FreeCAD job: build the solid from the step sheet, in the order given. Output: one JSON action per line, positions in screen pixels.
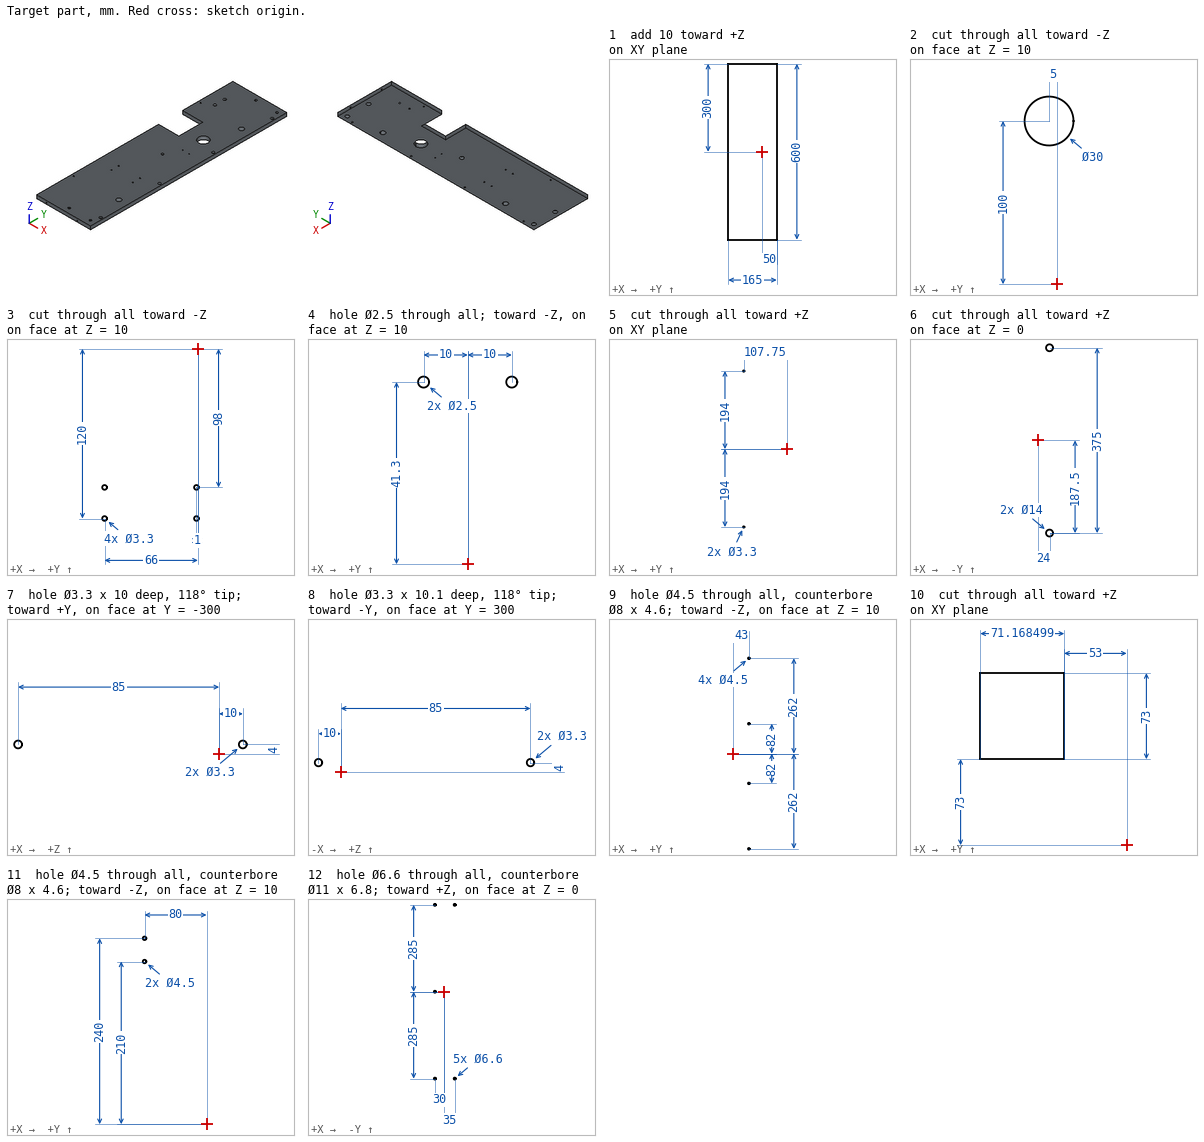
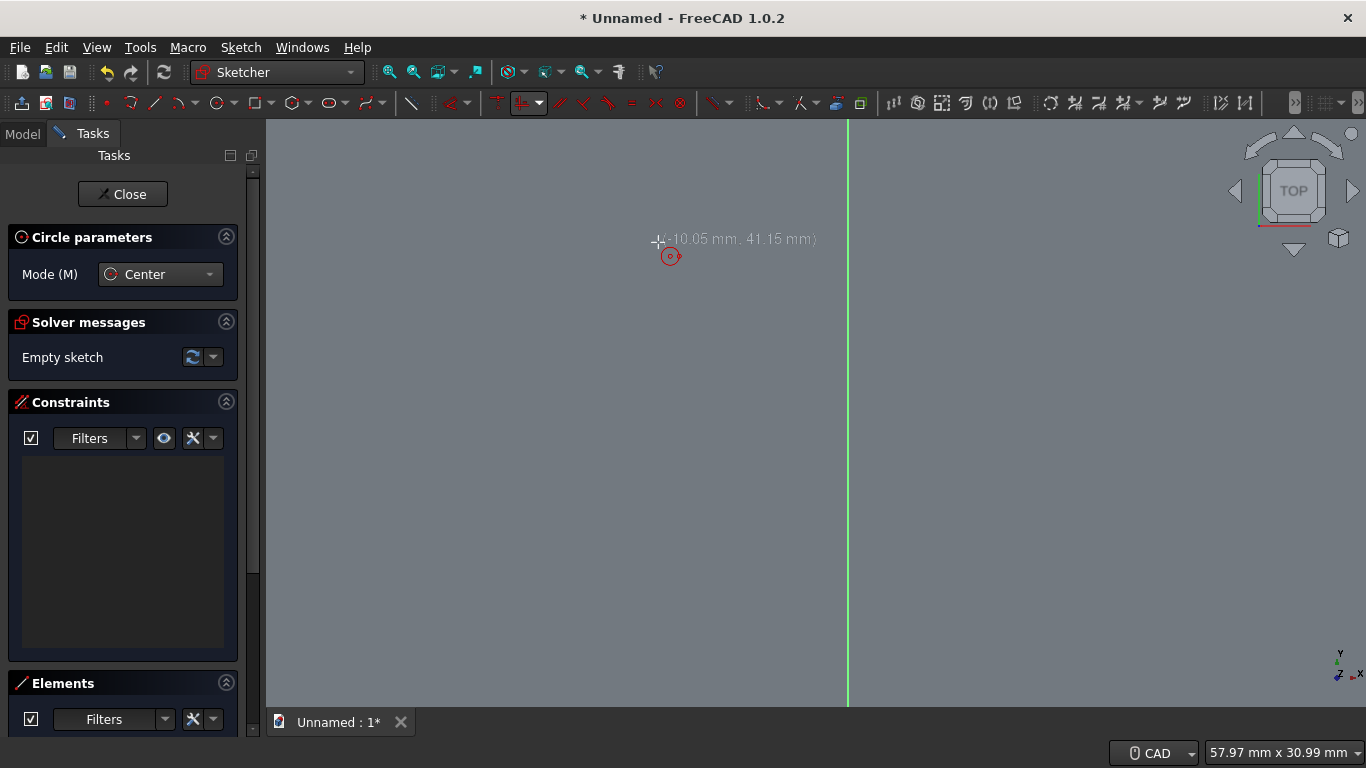
{"action": "left_click", "coordinate": [659, 241]}
{"action": "mouse_move", "coordinate": [675, 224]}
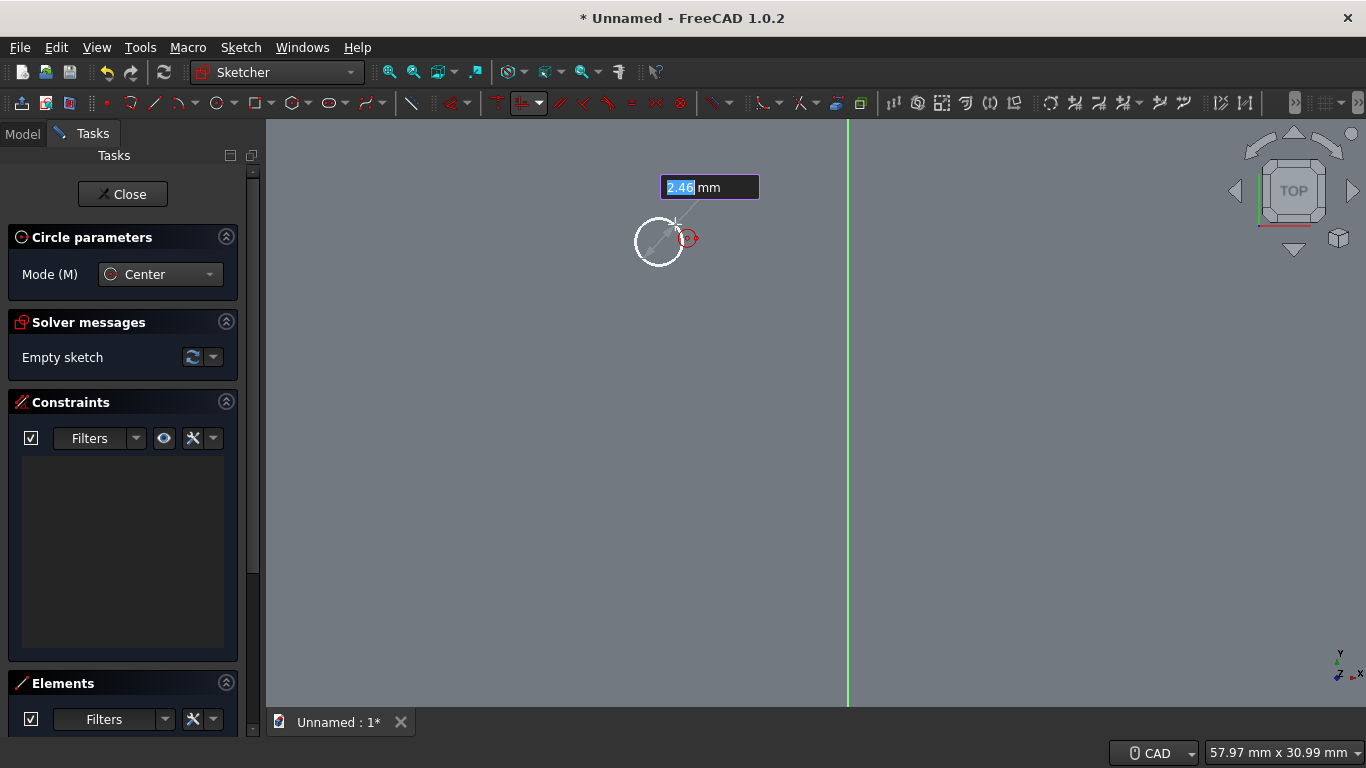
{"action": "type", "text": "2.5"}
{"action": "key", "text": "Return"}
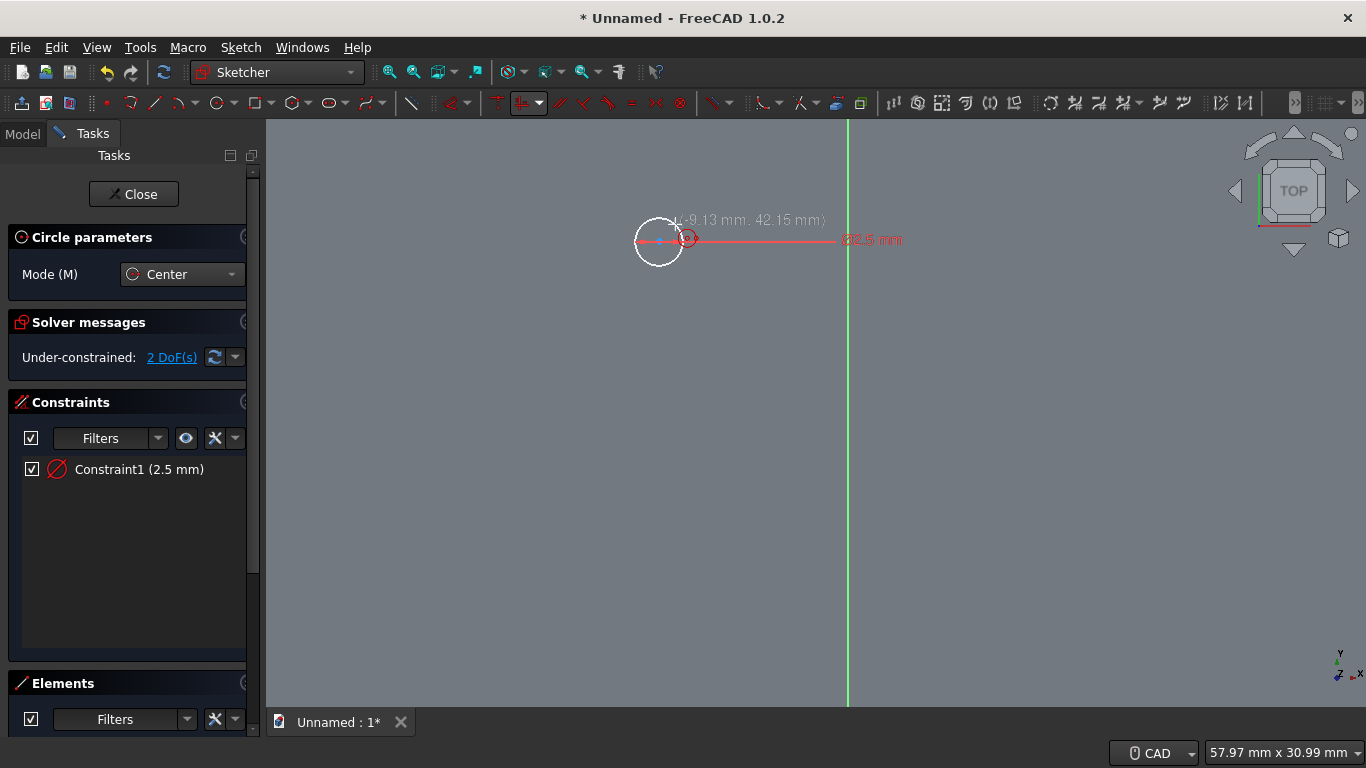
{"action": "left_click", "coordinate": [1038, 241]}
{"action": "mouse_move", "coordinate": [1055, 224]}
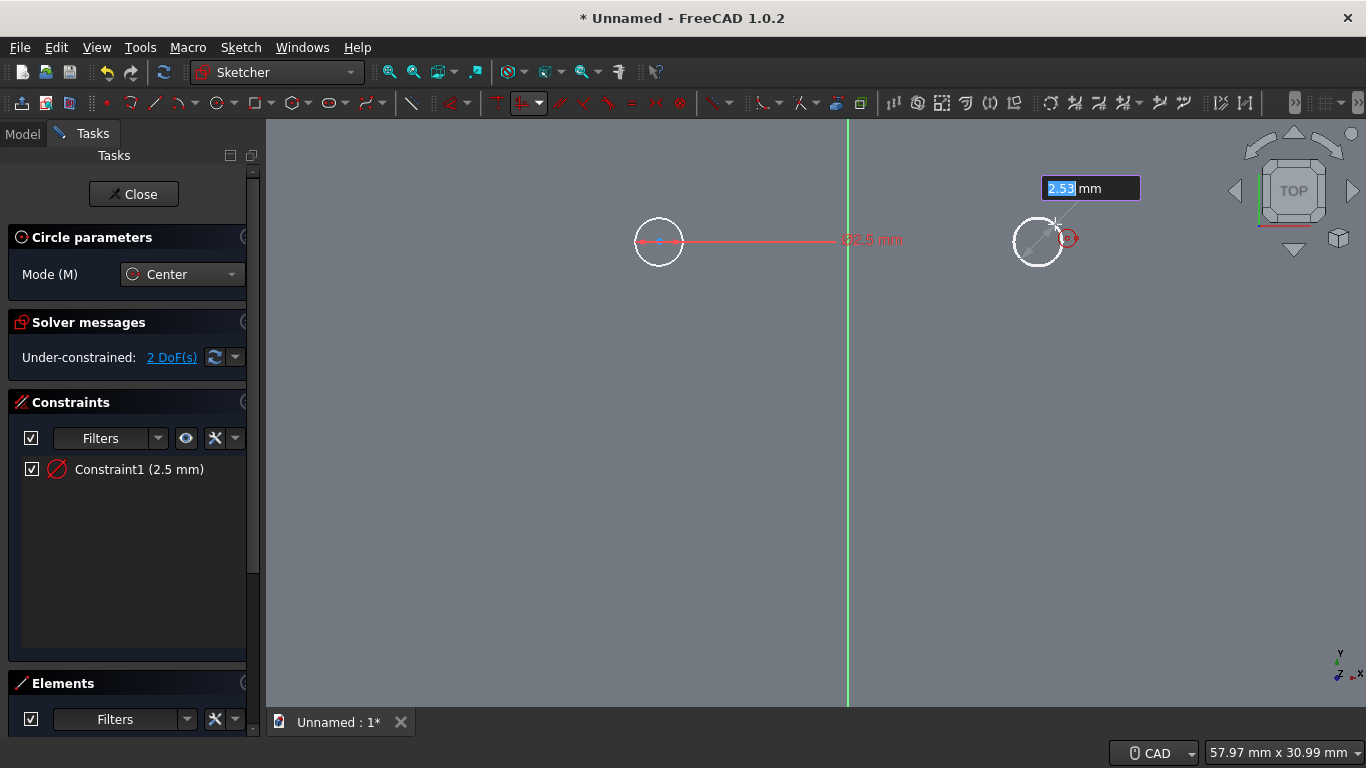
{"action": "type", "text": "2.5"}
{"action": "key", "text": "Return"}
{"action": "key", "text": "Escape"}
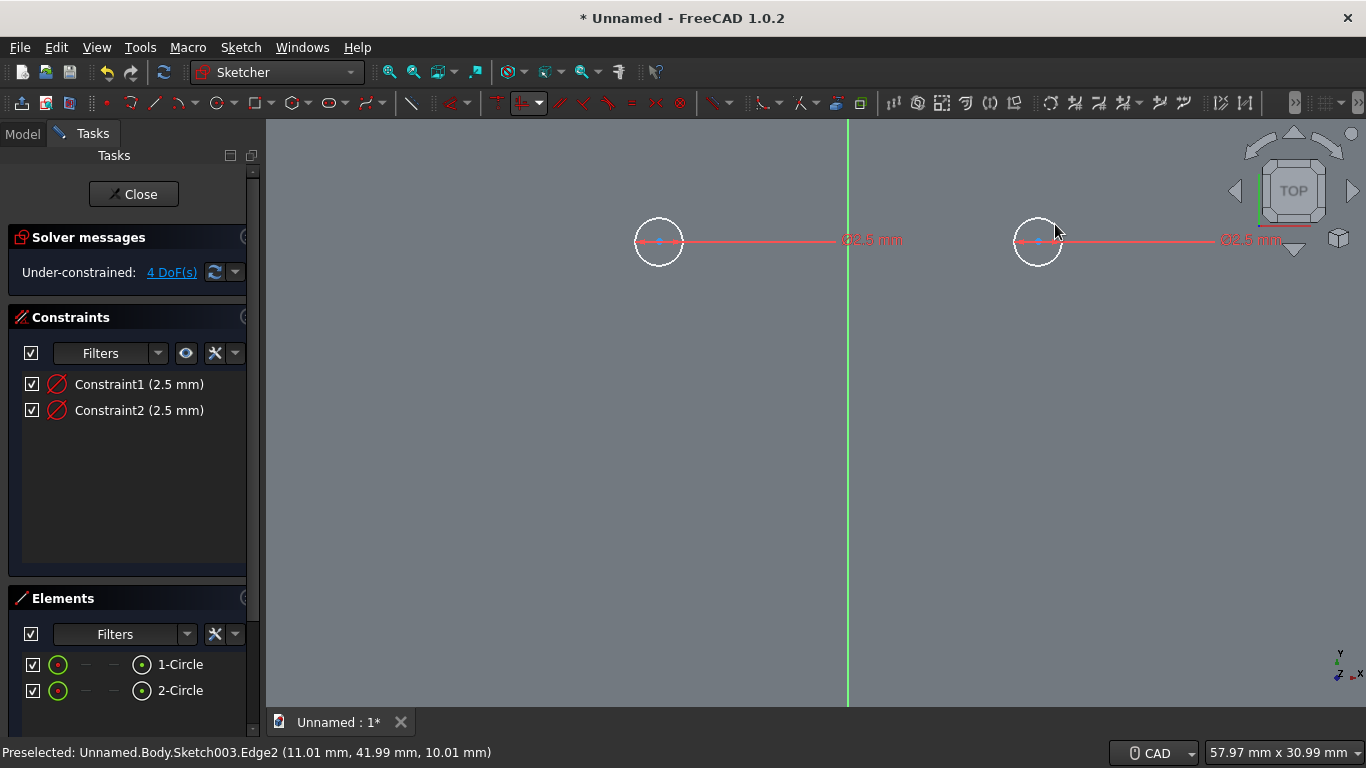
{"action": "left_click", "coordinate": [659, 242]}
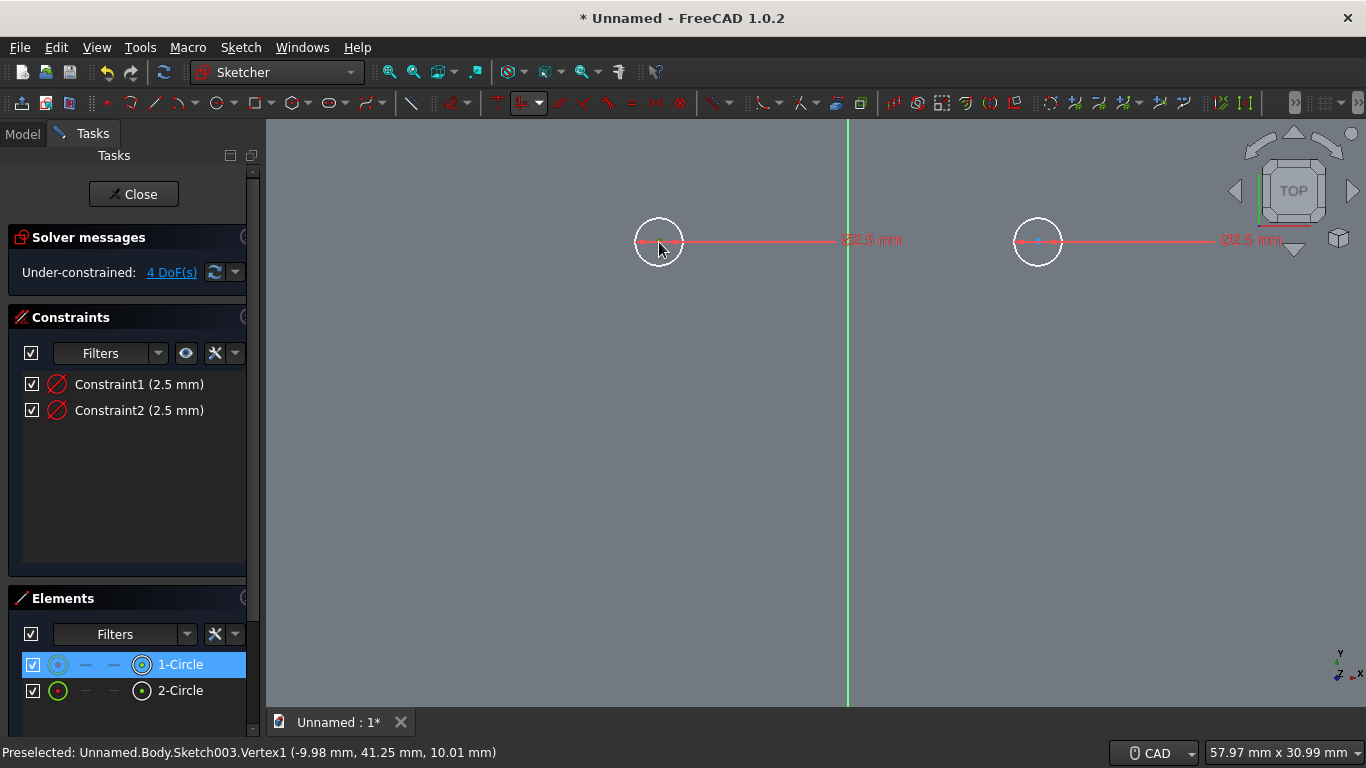
{"action": "left_click", "coordinate": [1038, 242]}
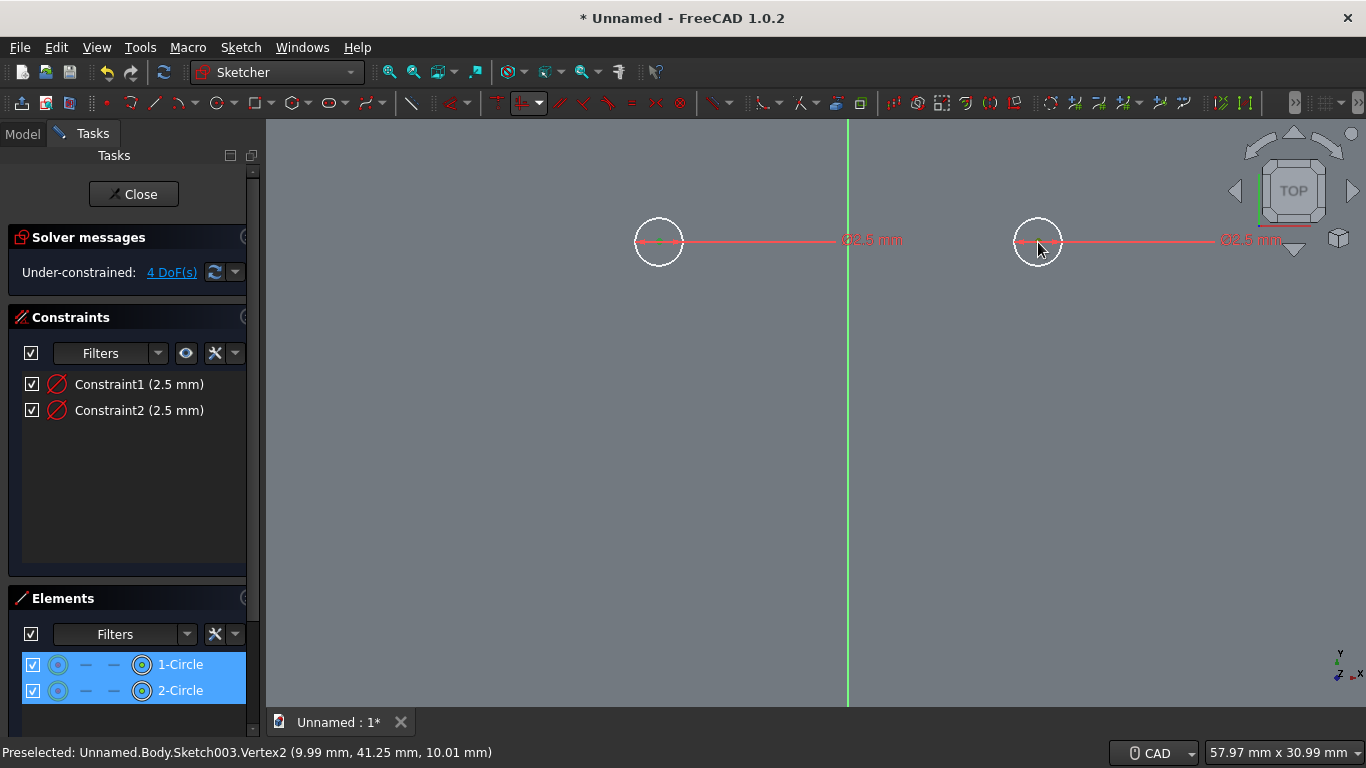
{"action": "left_click", "coordinate": [542, 104]}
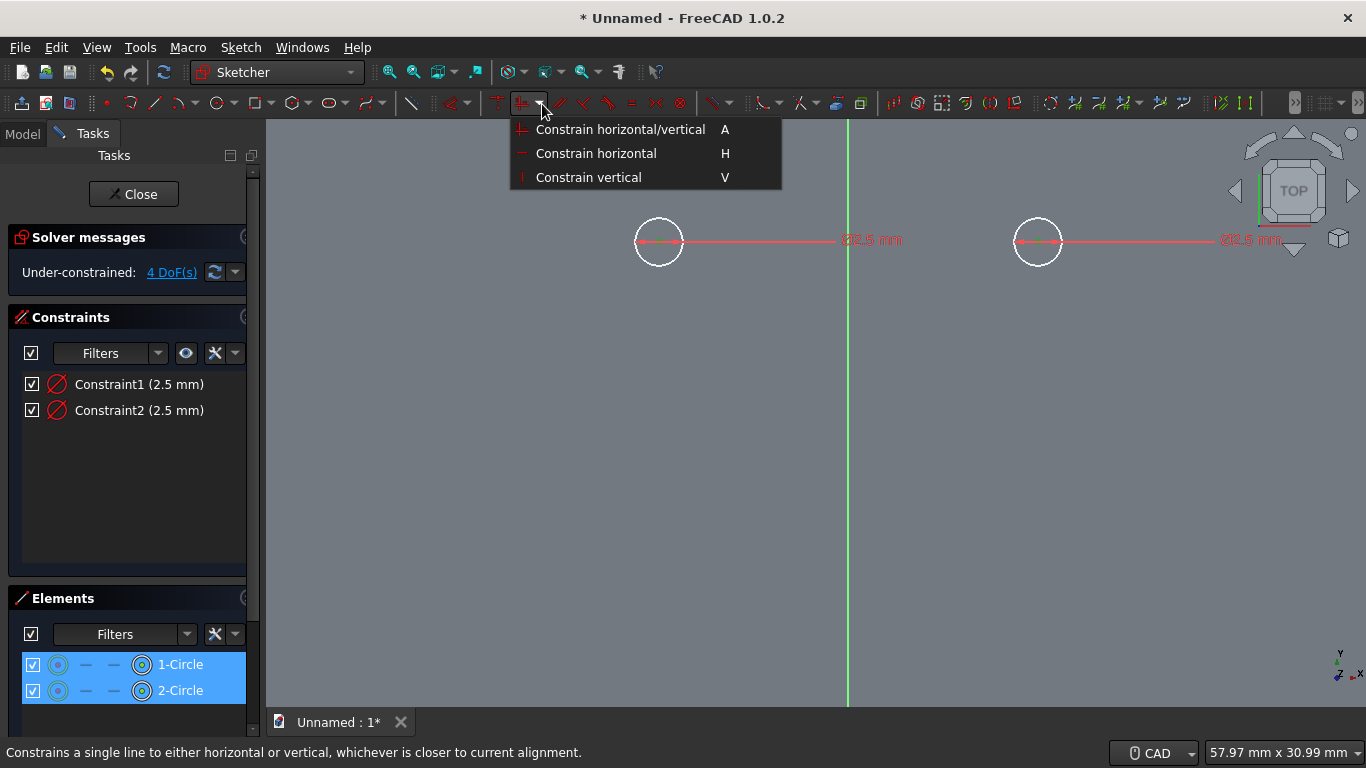
{"action": "left_click", "coordinate": [646, 153]}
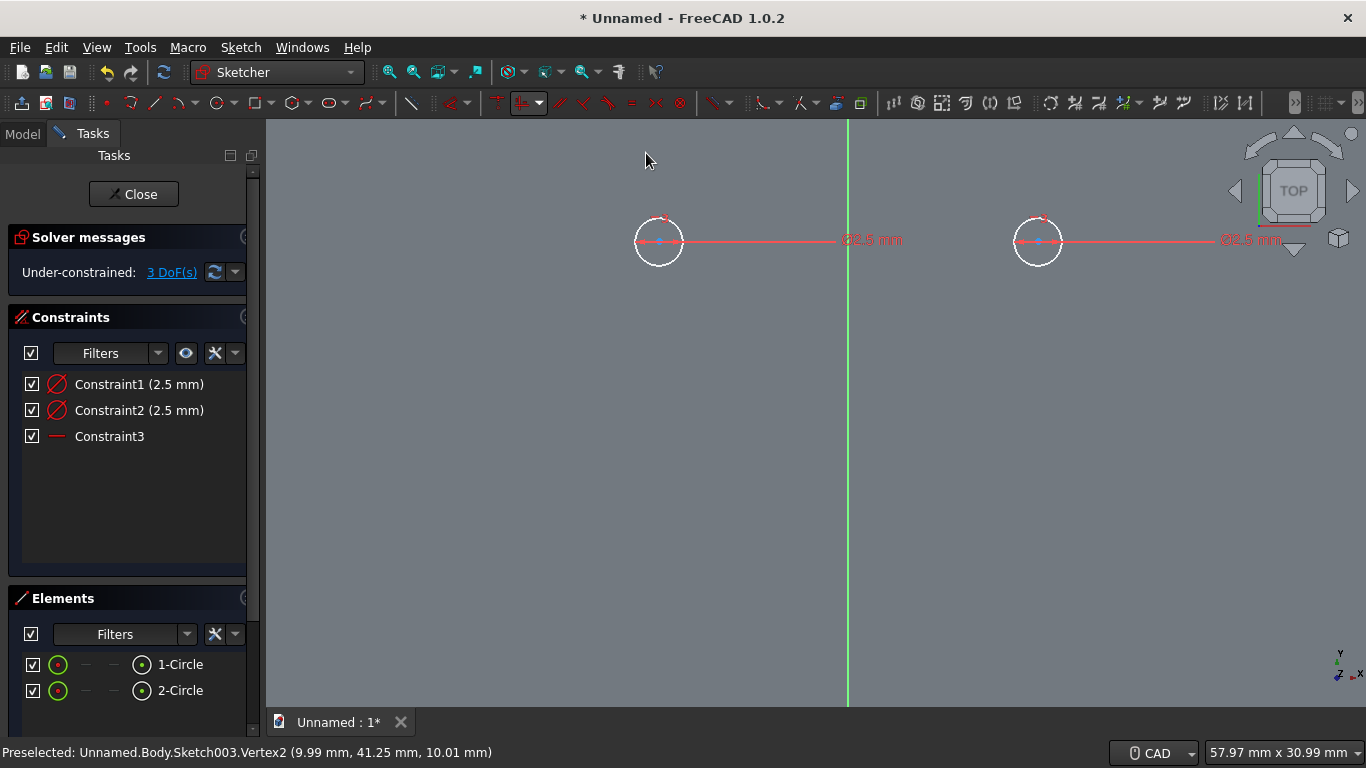
{"action": "key", "text": "d"}